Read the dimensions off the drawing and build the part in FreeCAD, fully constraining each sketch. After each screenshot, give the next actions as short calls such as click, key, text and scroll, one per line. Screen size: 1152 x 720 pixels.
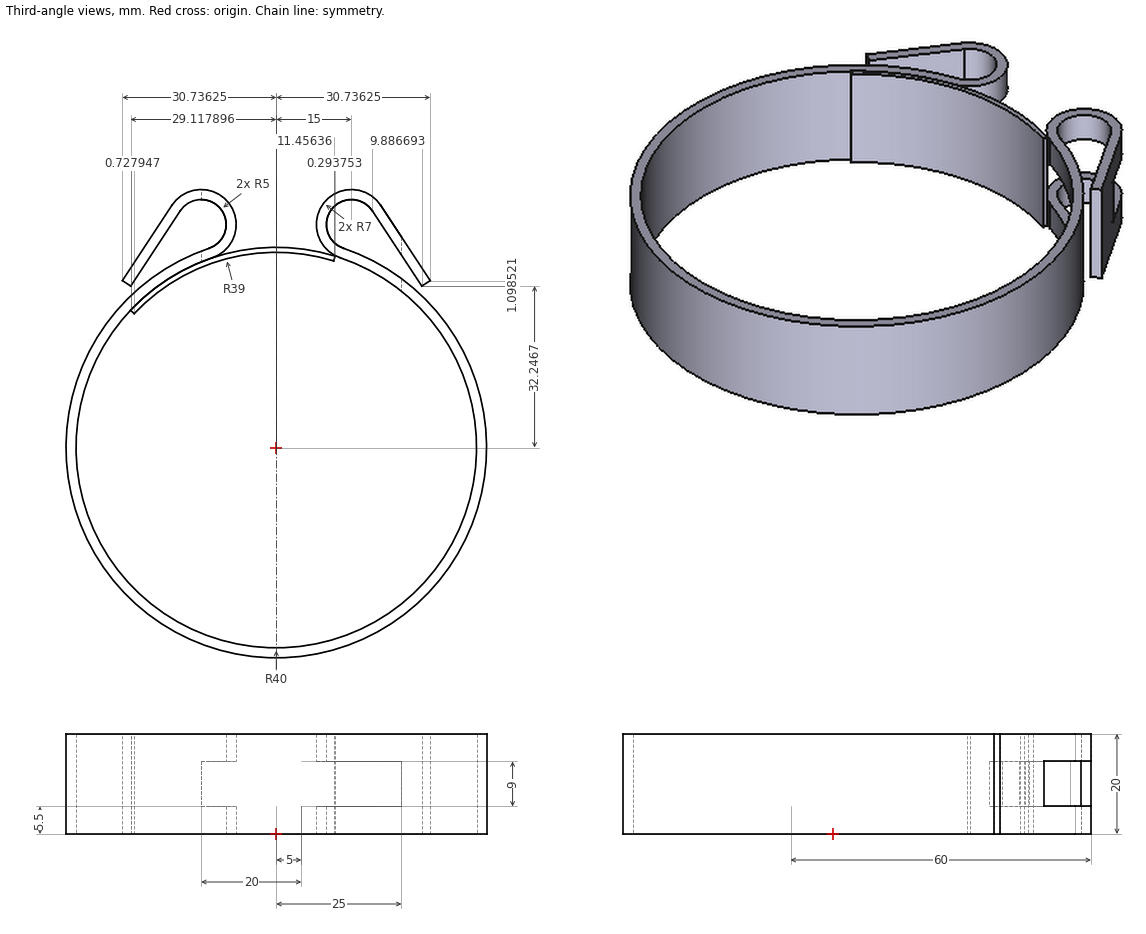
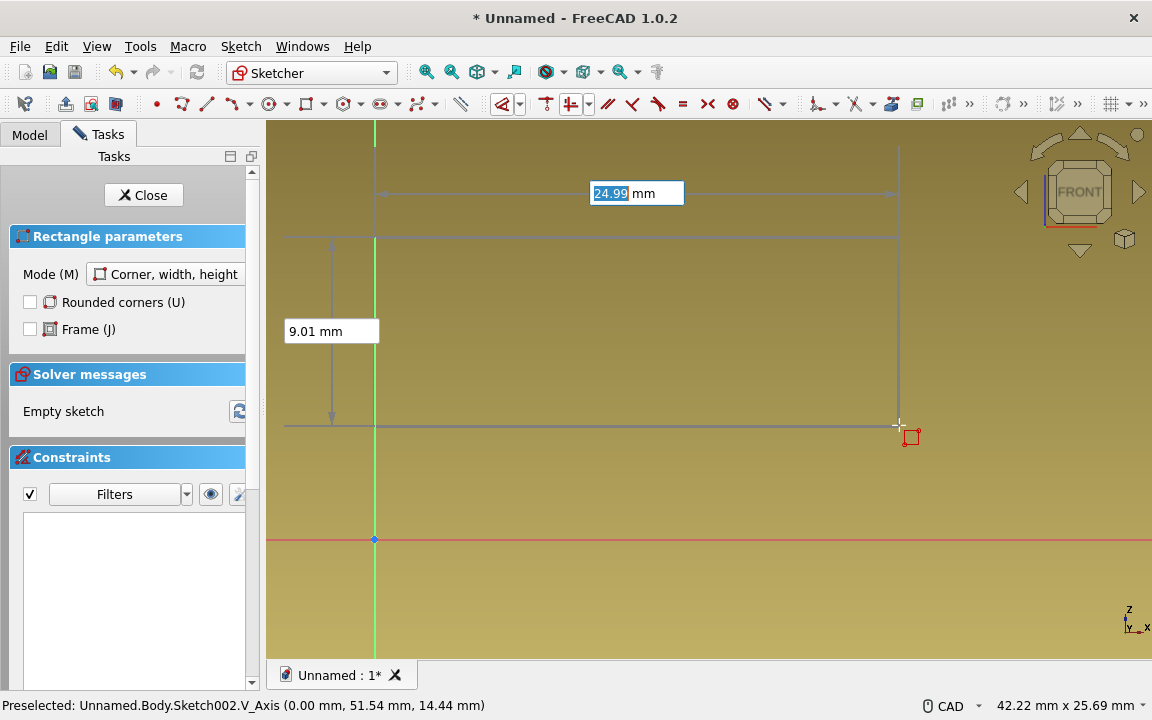
text(25)
key(Tab)
text(9)
key(Return)
key(Escape)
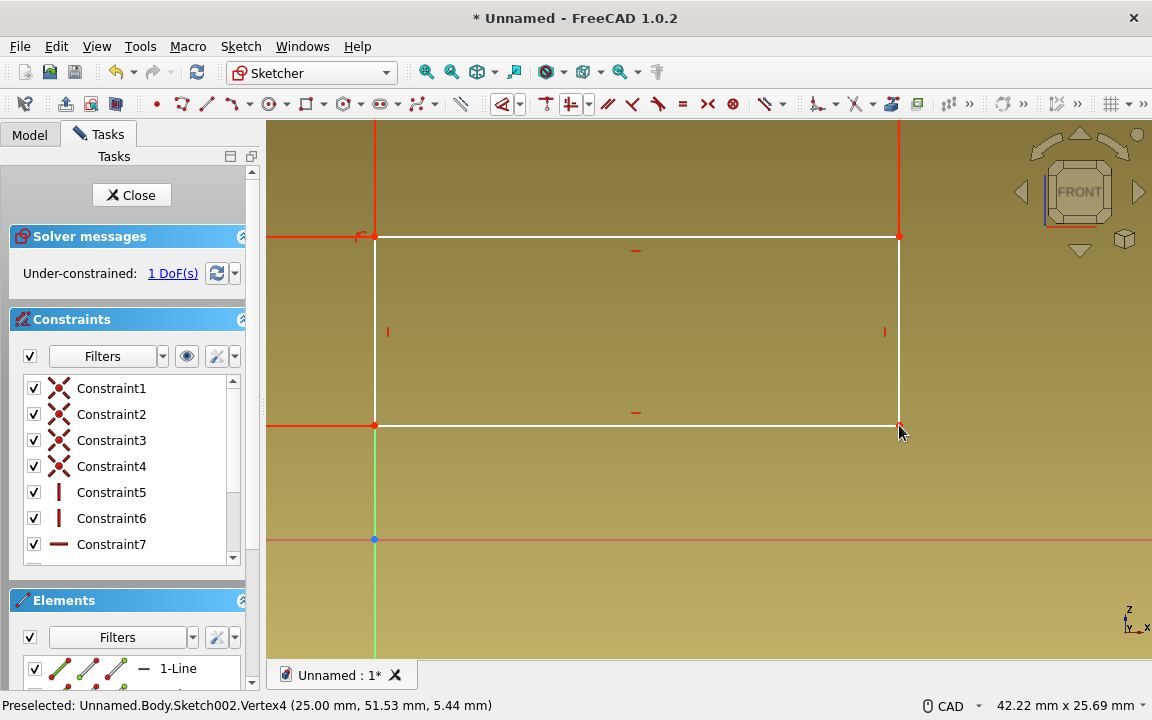
click(375, 426)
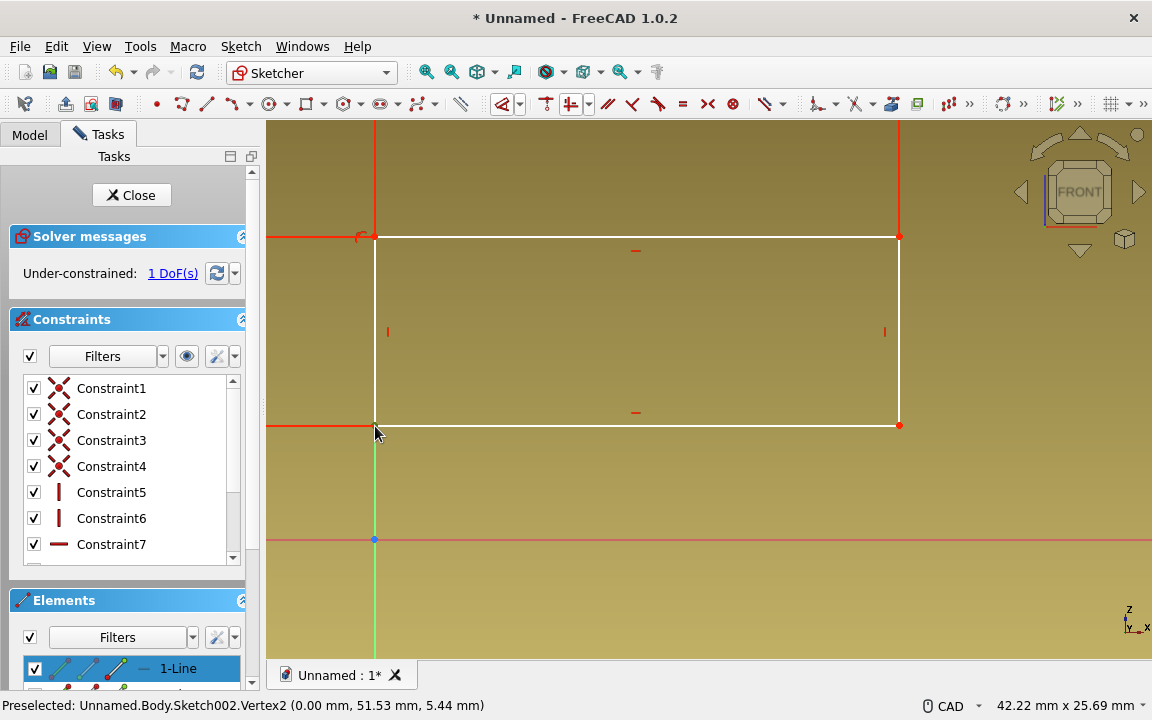
key(i)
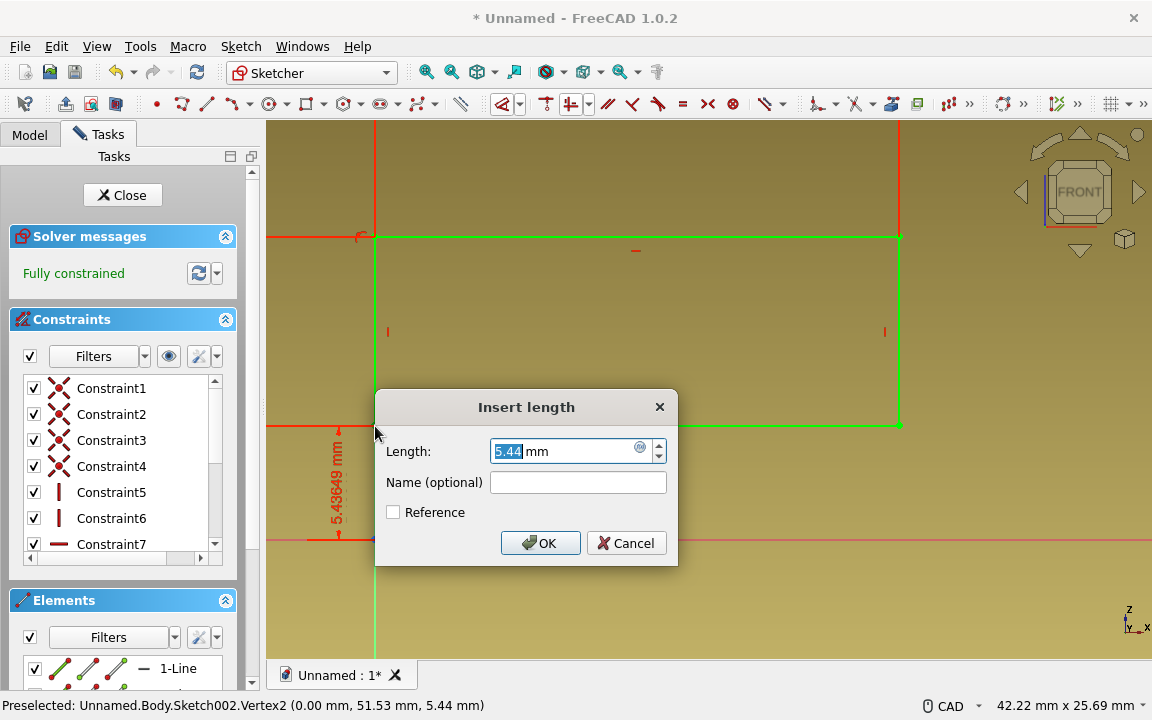
text(5.5)
key(Return)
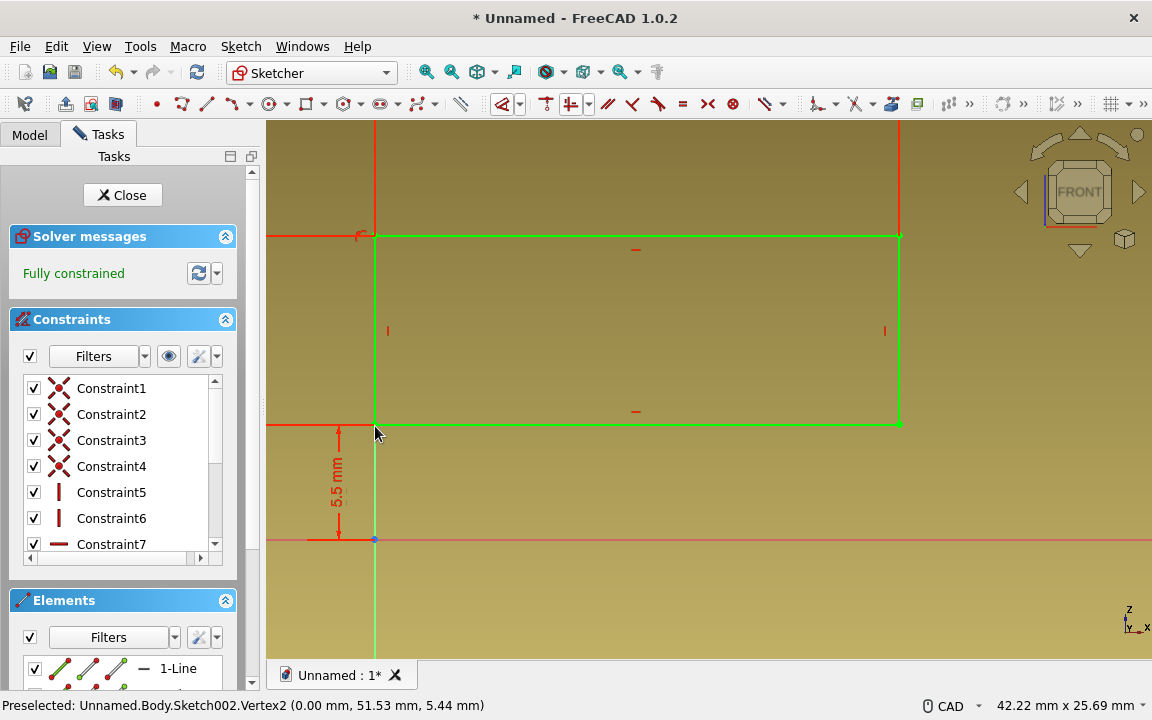
click(123, 195)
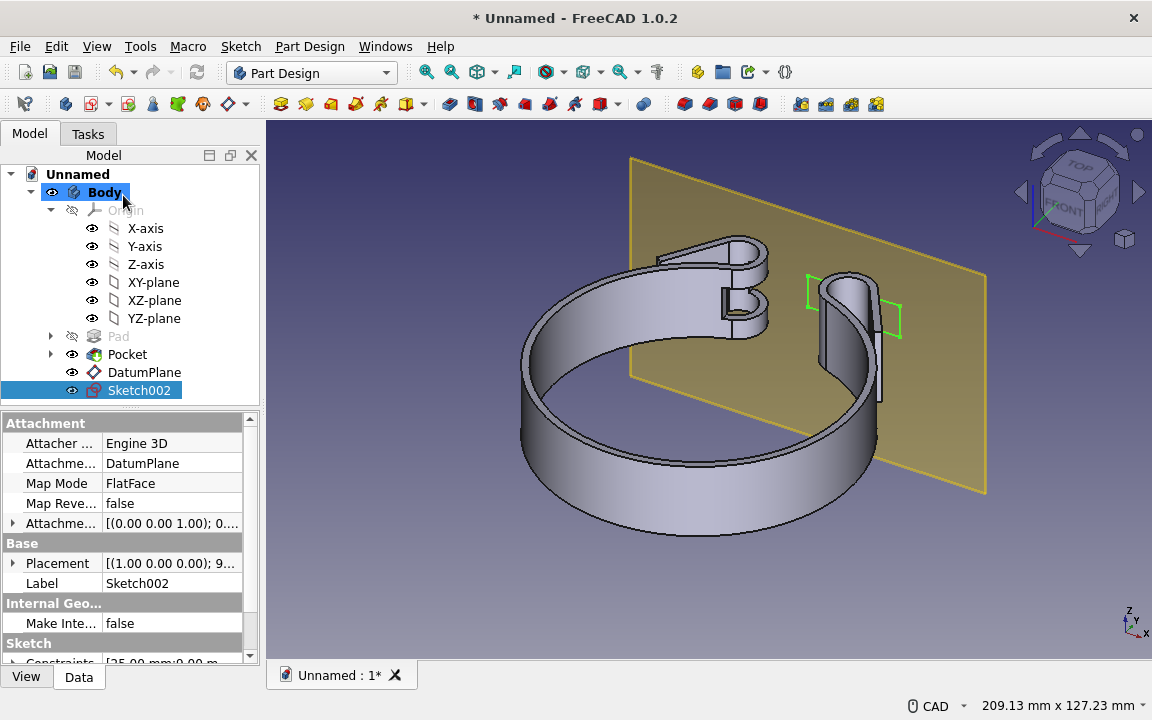
click(450, 104)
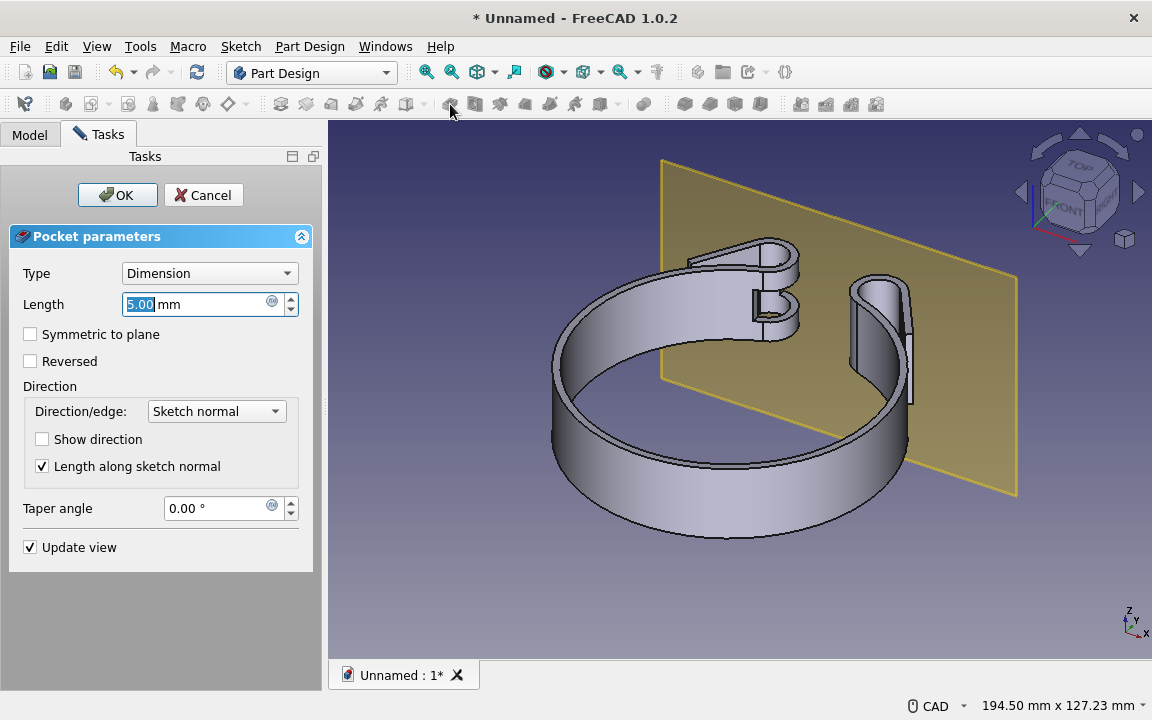
text(60)
key(Tab)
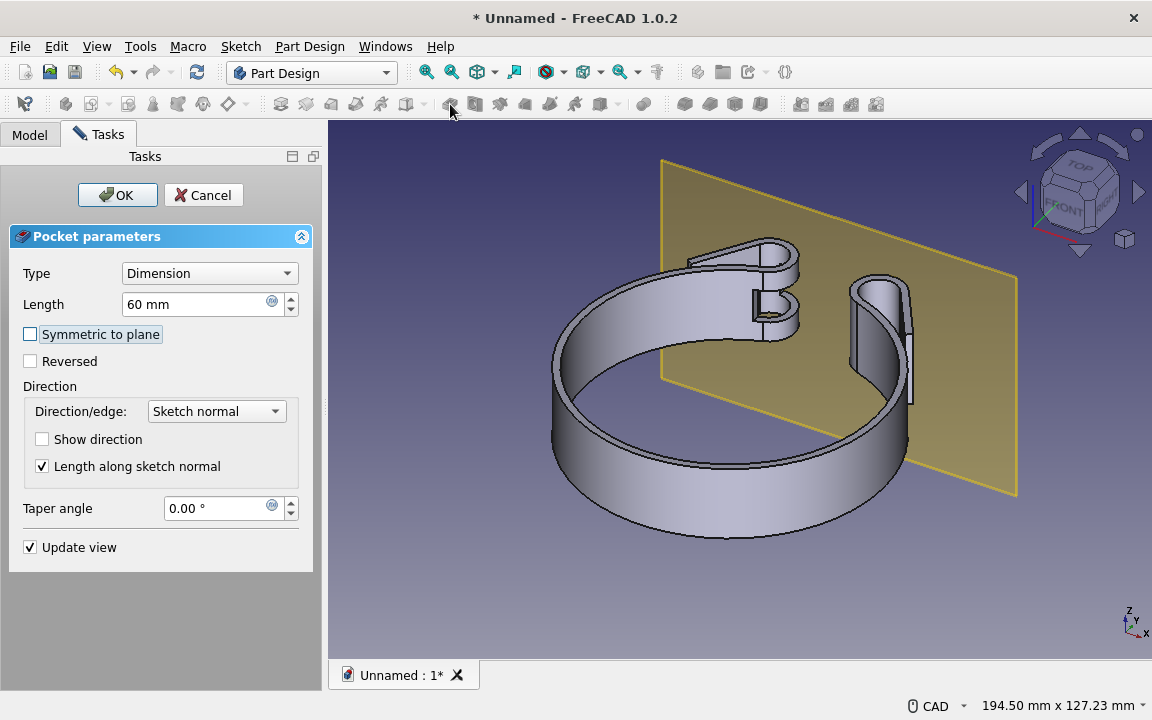
click(31, 361)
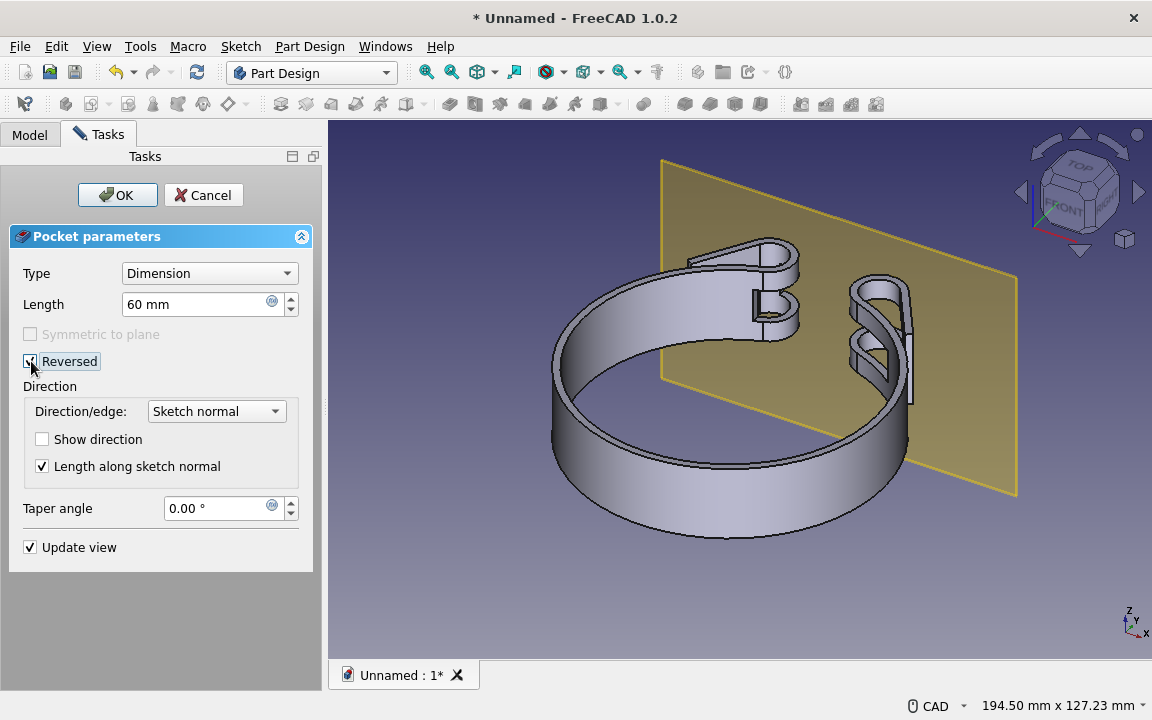
click(118, 195)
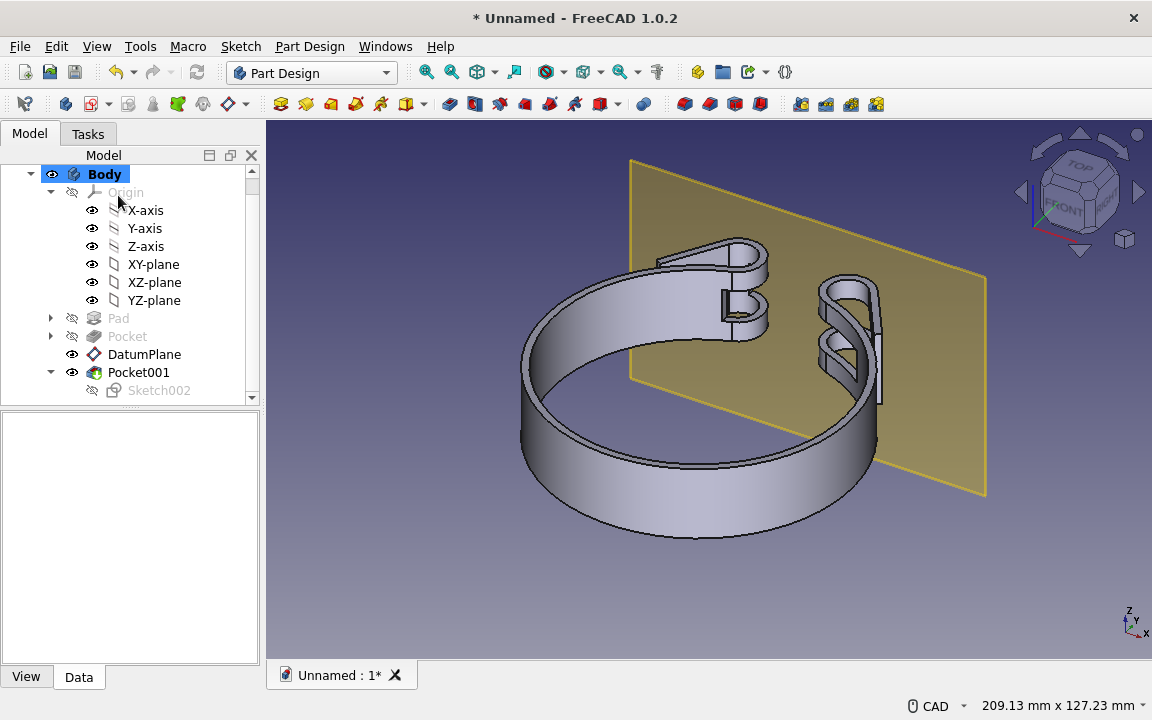
click(117, 354)
key(space)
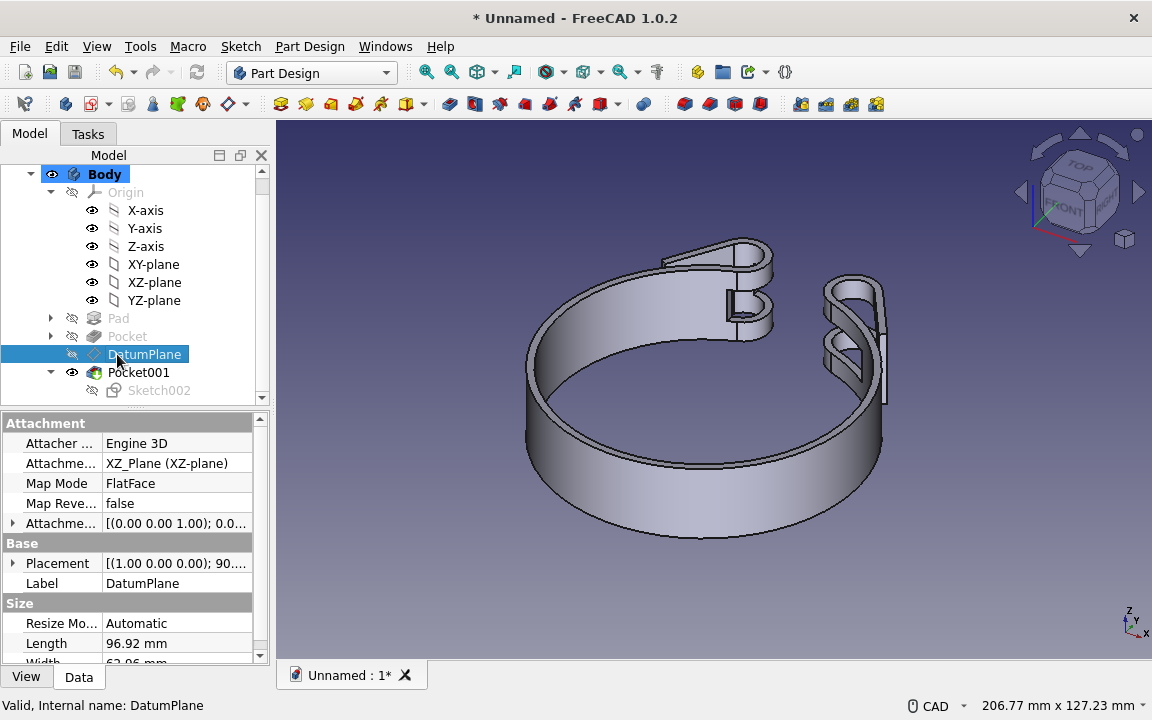
click(316, 619)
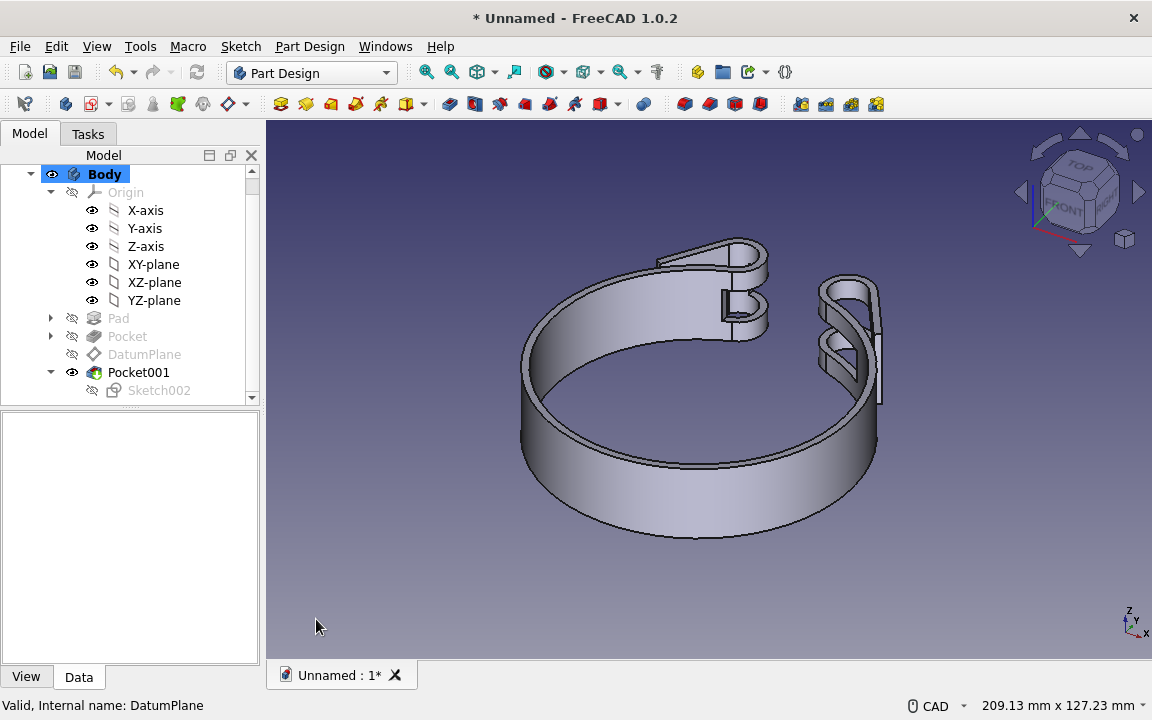
click(66, 104)